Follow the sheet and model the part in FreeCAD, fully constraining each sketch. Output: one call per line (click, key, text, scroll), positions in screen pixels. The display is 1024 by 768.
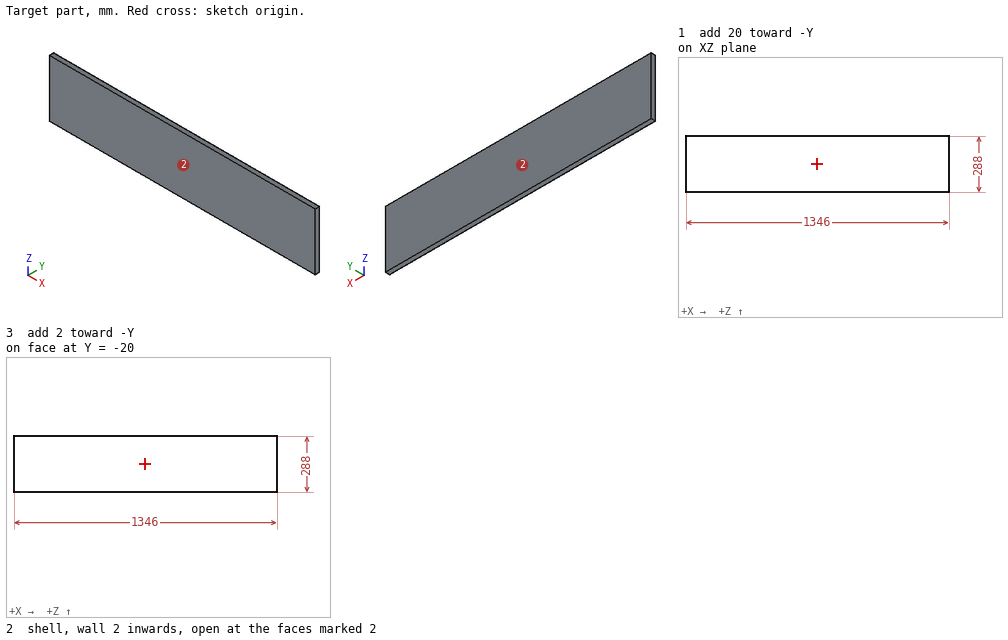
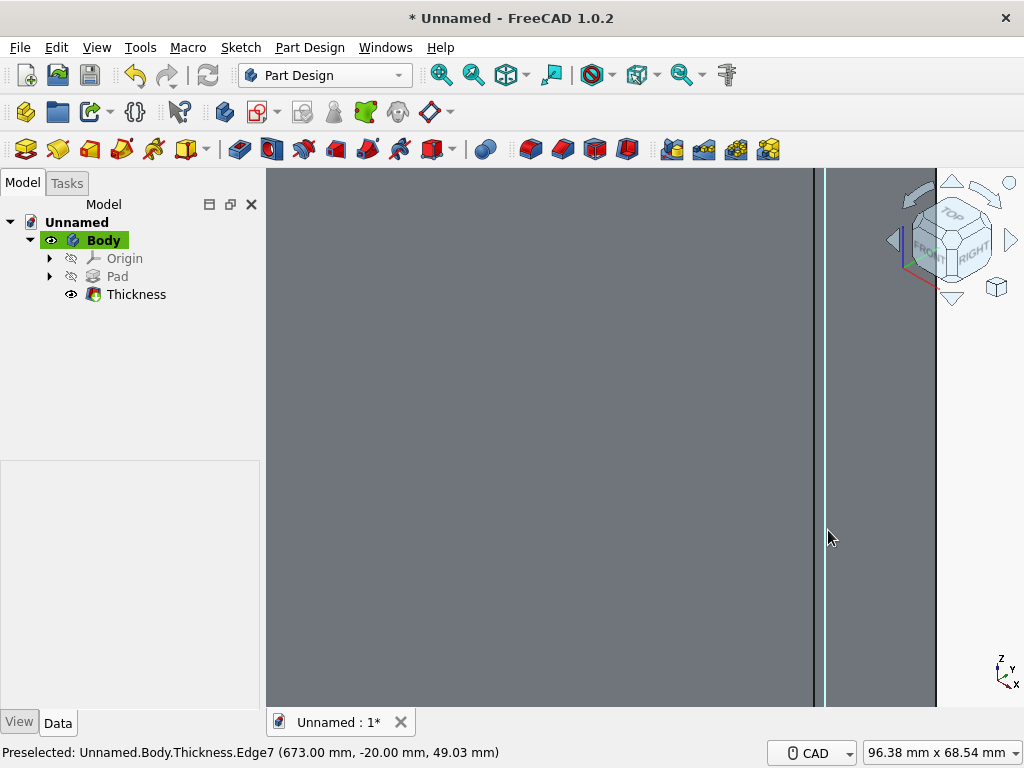
scroll(818, 539, up, 5)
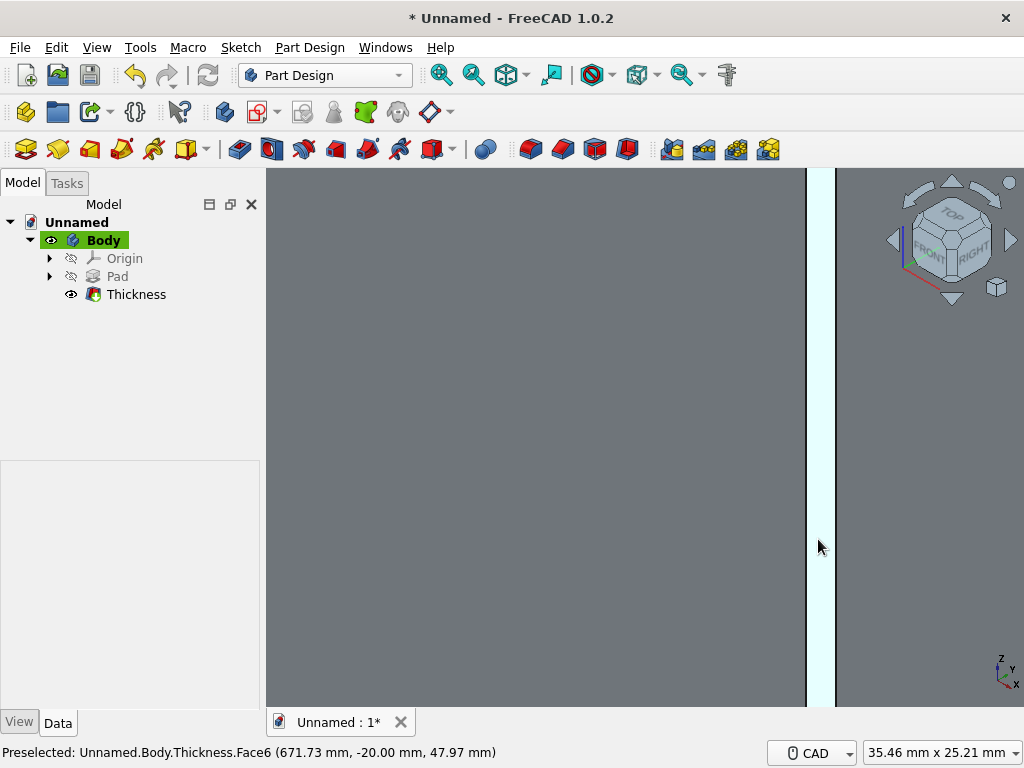
click(816, 538)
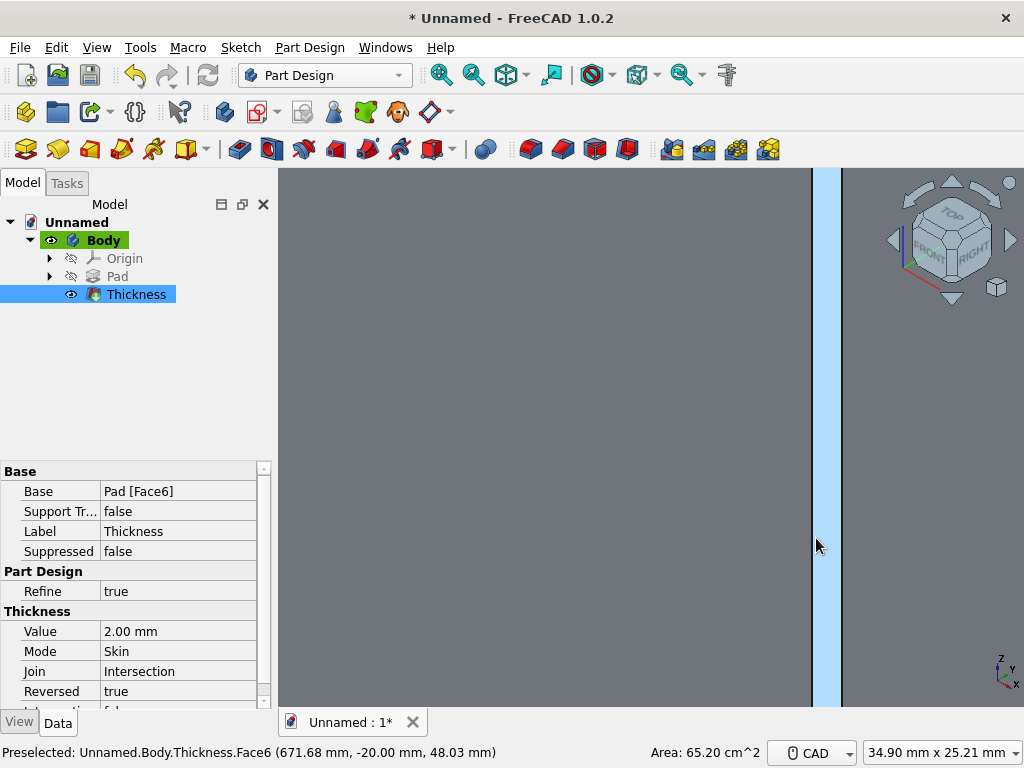
click(258, 112)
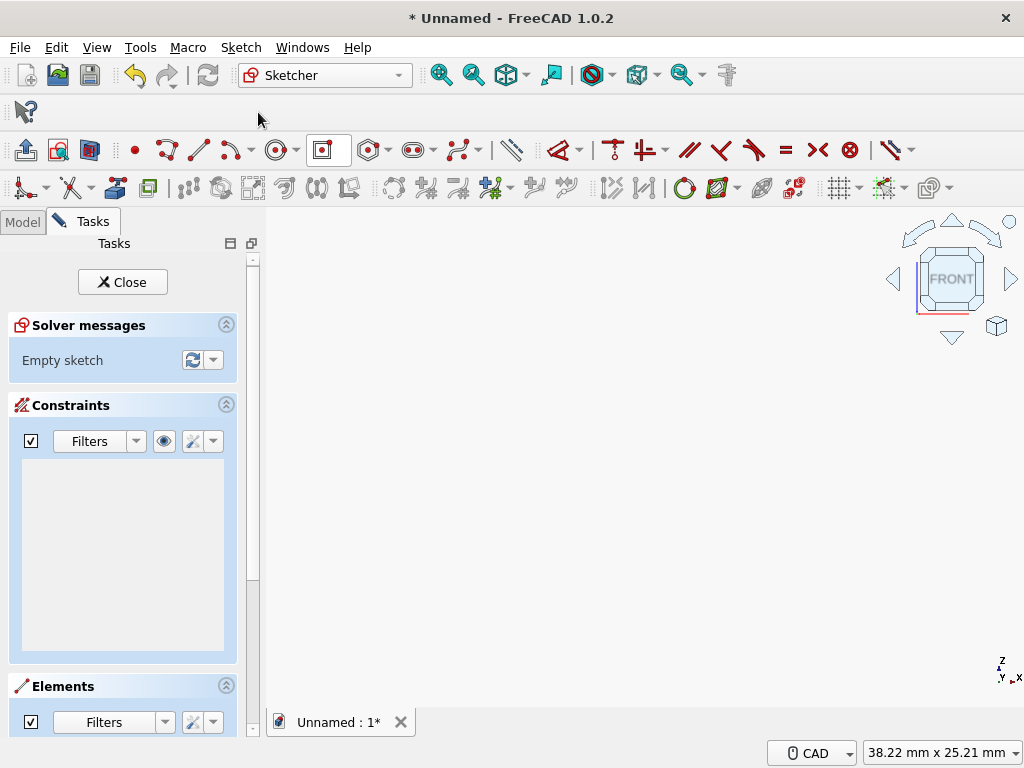
scroll(576, 457, down, 15)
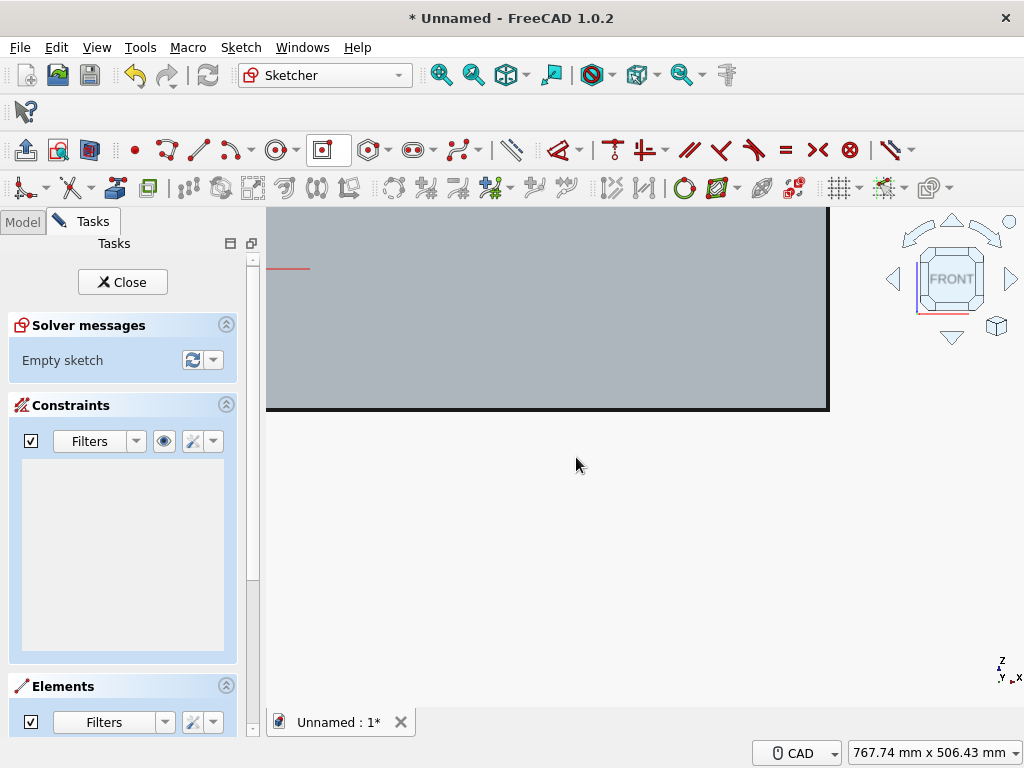
scroll(754, 538, down, 6)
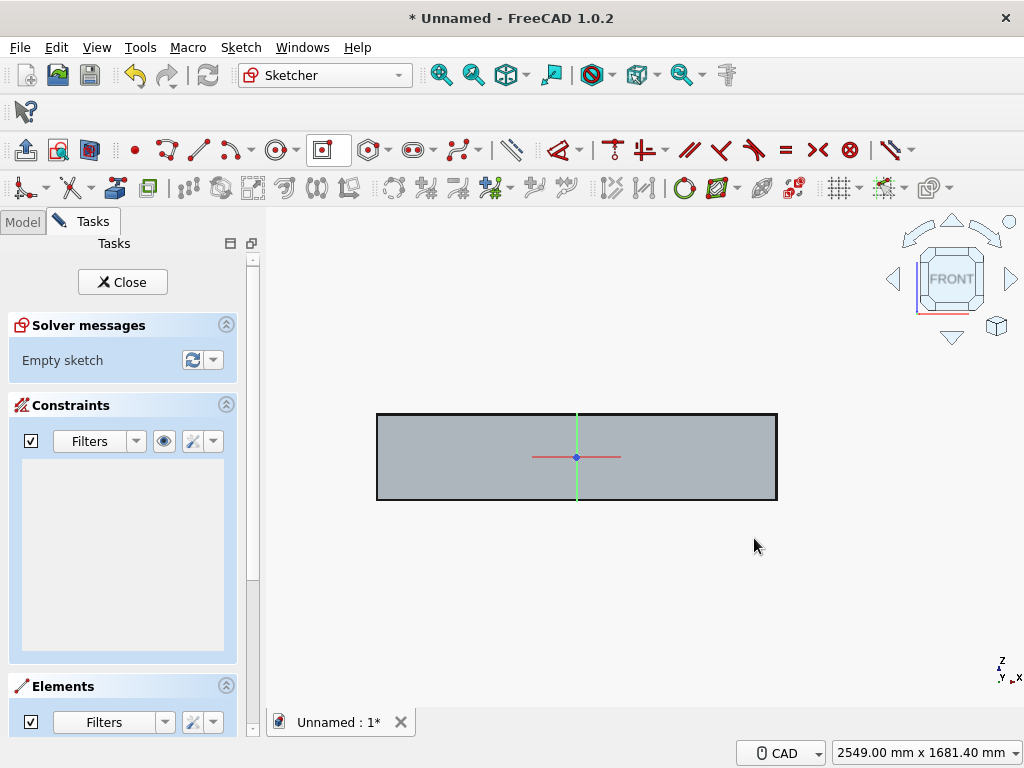
key(g)
key(v)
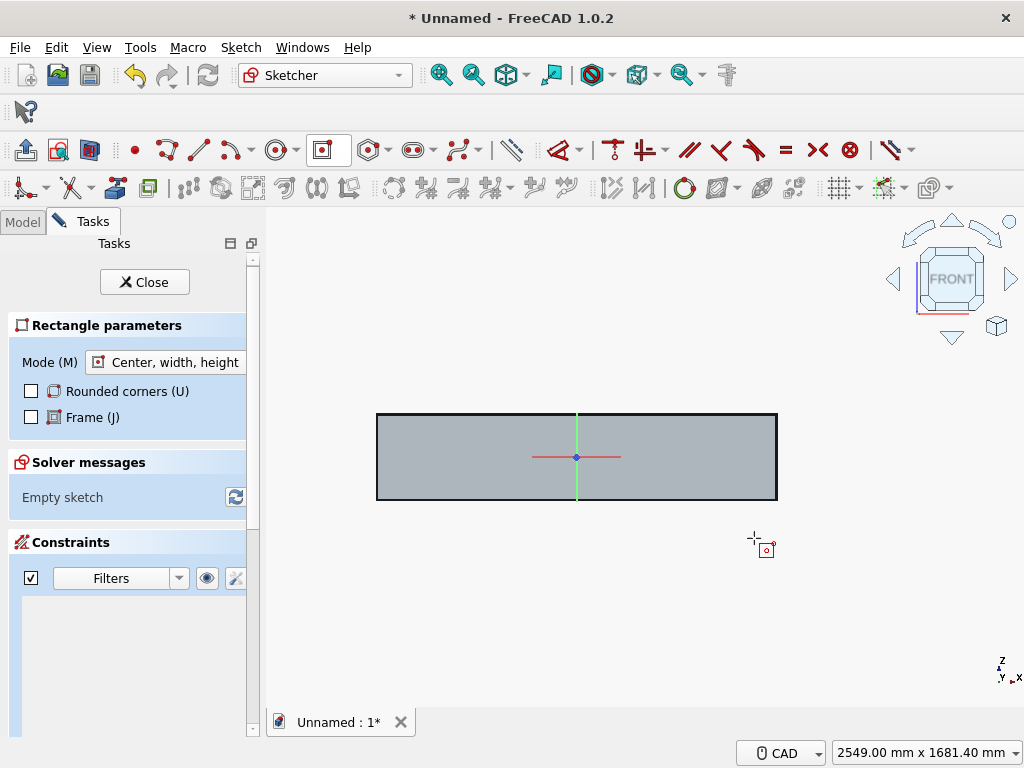
click(577, 457)
click(777, 414)
key(Escape)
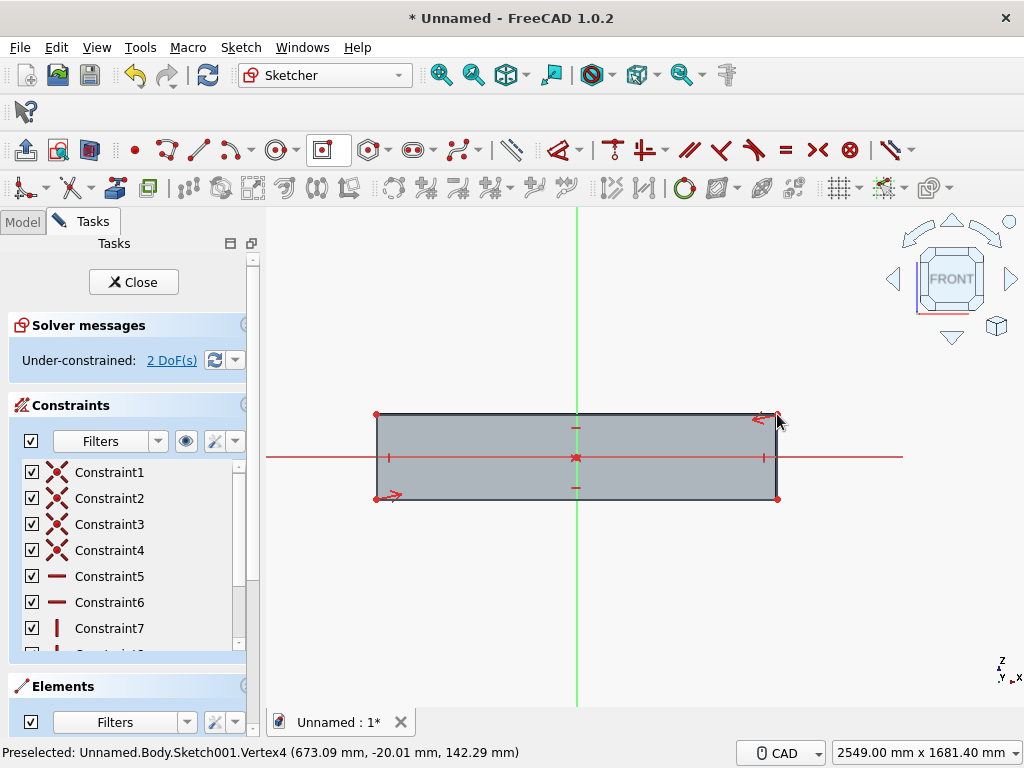
key(d)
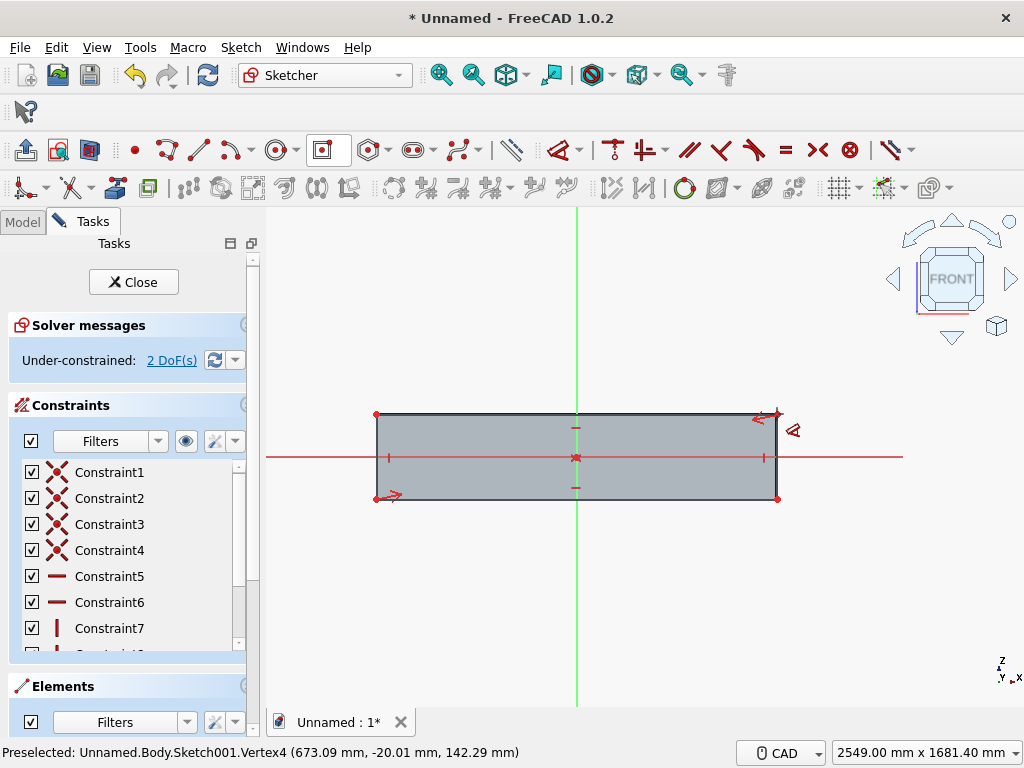
click(777, 474)
click(811, 438)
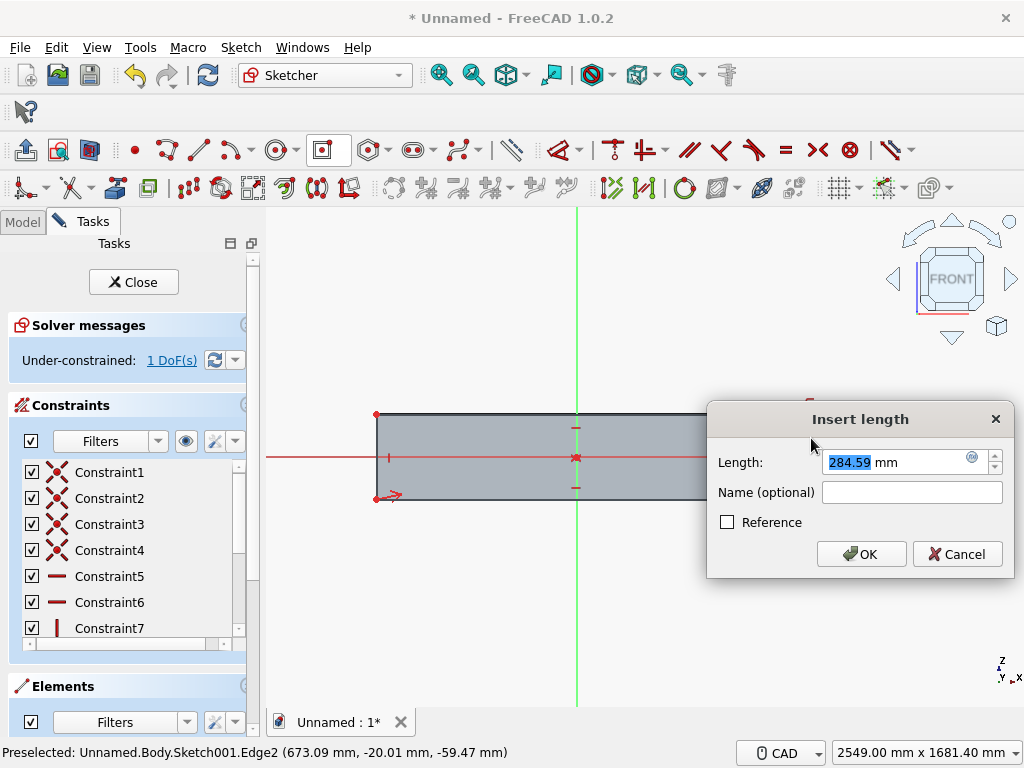
text(288)
key(Return)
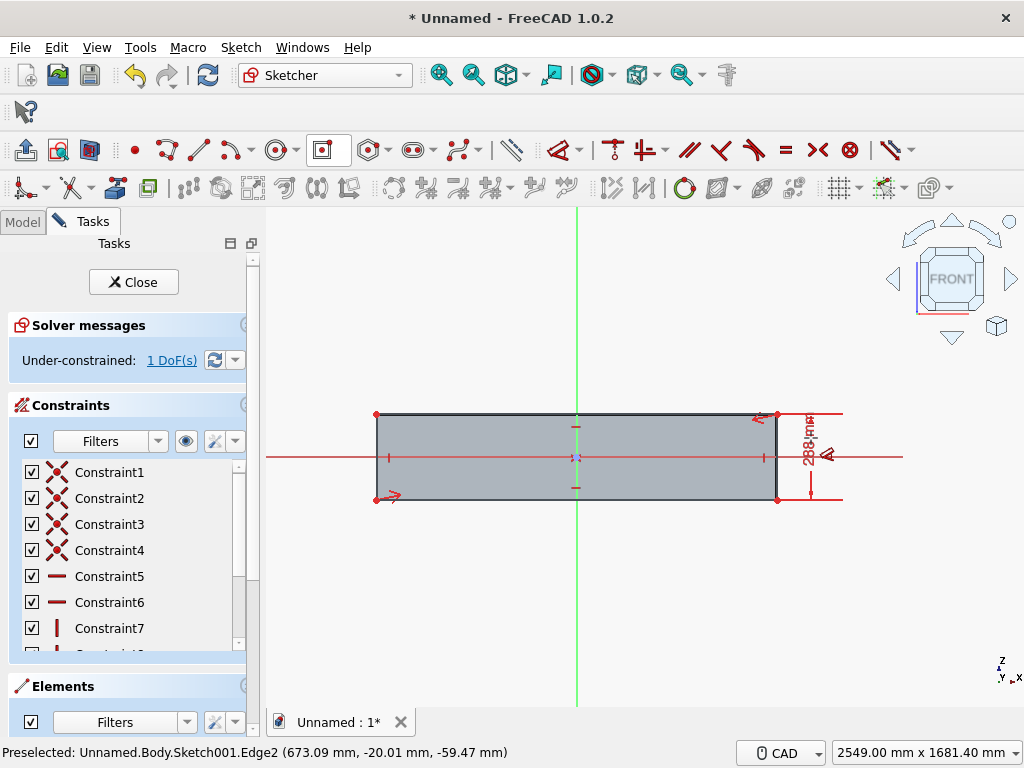
click(497, 500)
click(485, 534)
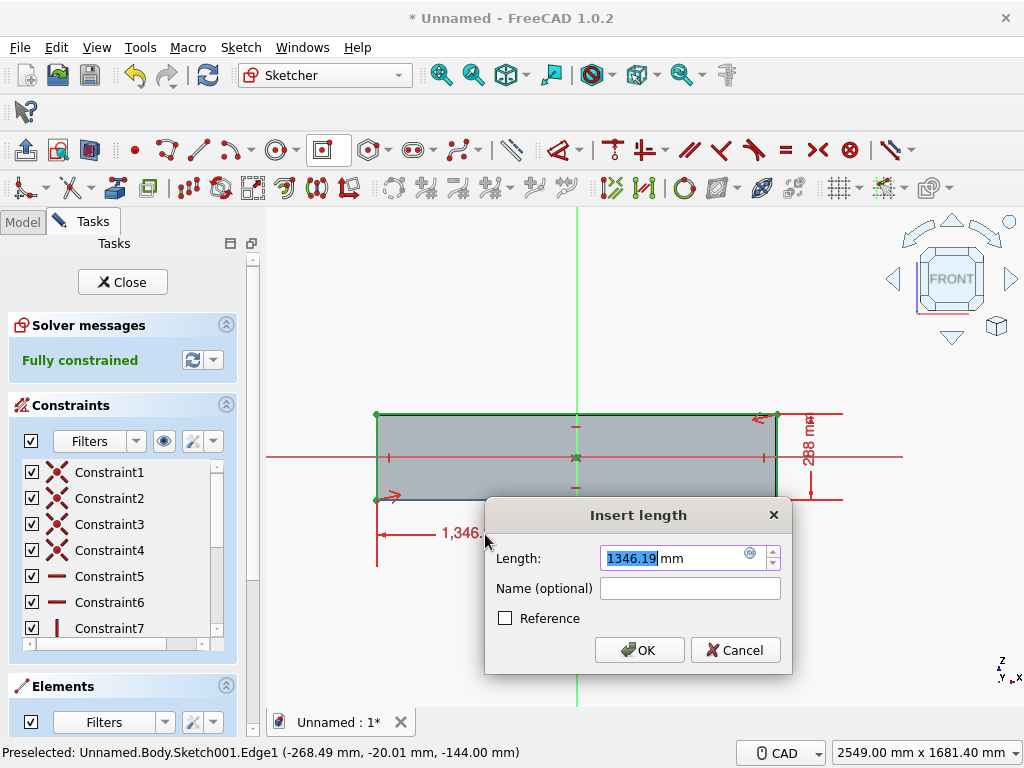
text(1346)
key(Return)
key(Escape)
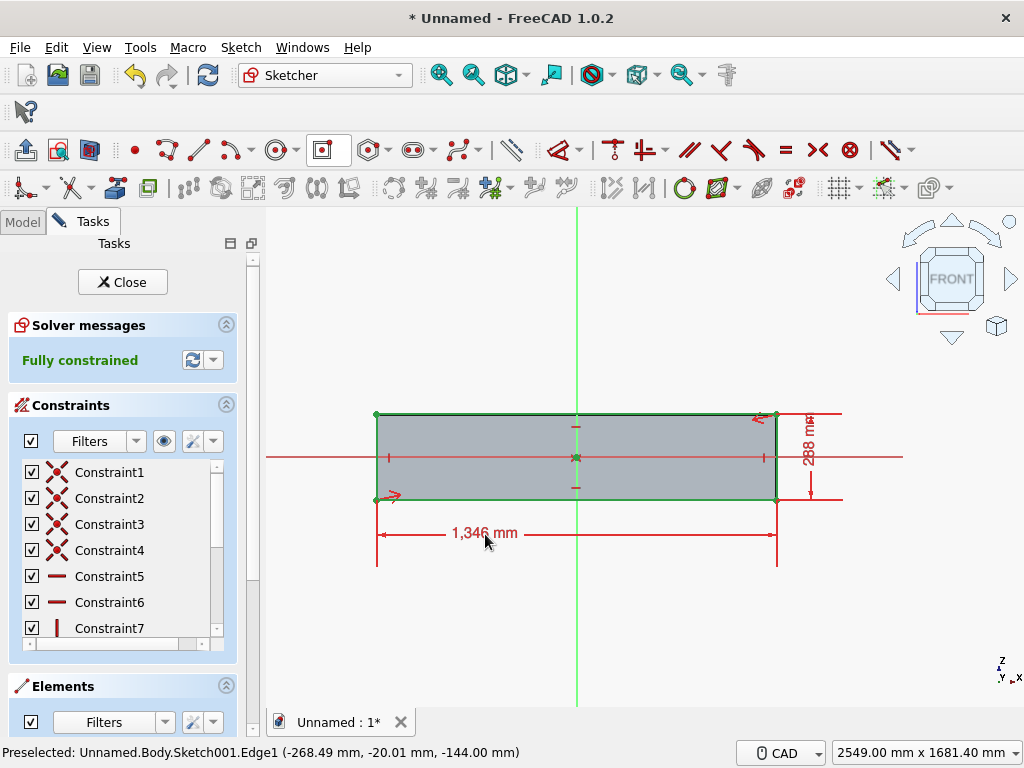
click(123, 282)